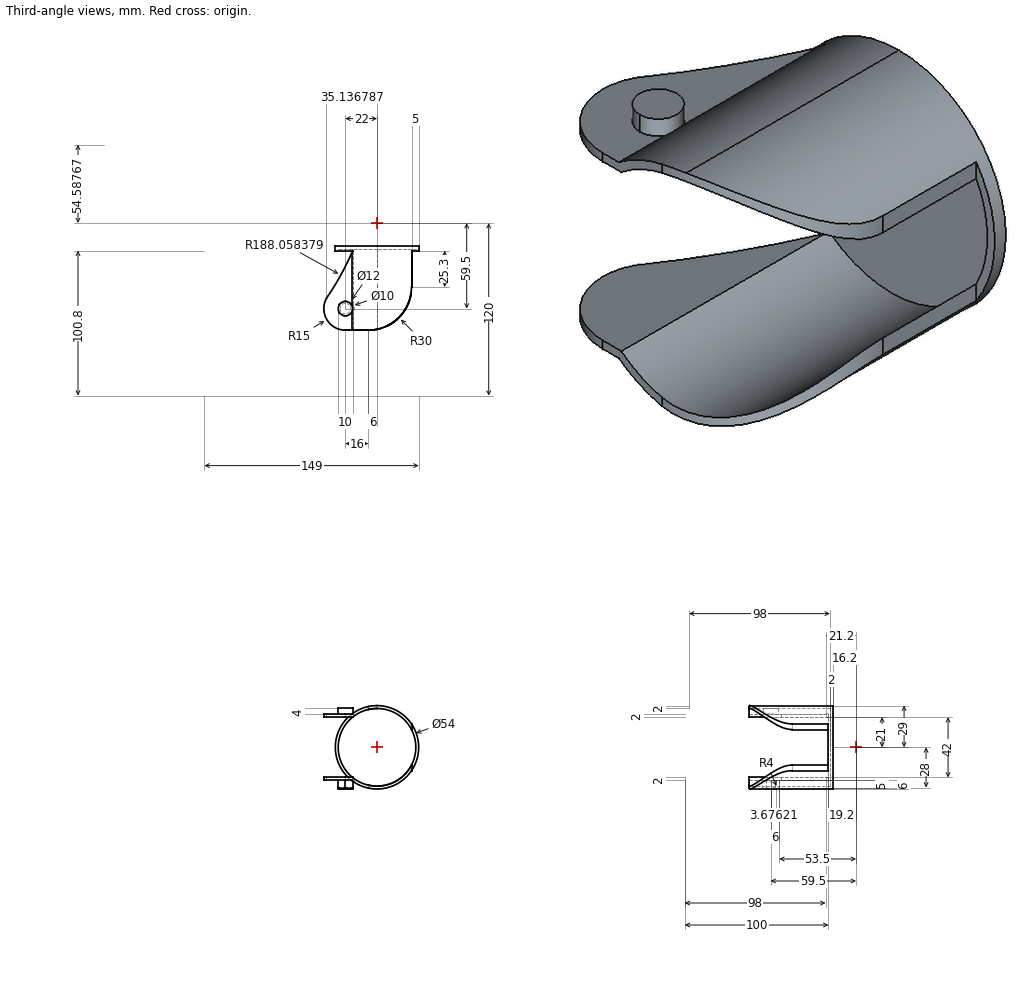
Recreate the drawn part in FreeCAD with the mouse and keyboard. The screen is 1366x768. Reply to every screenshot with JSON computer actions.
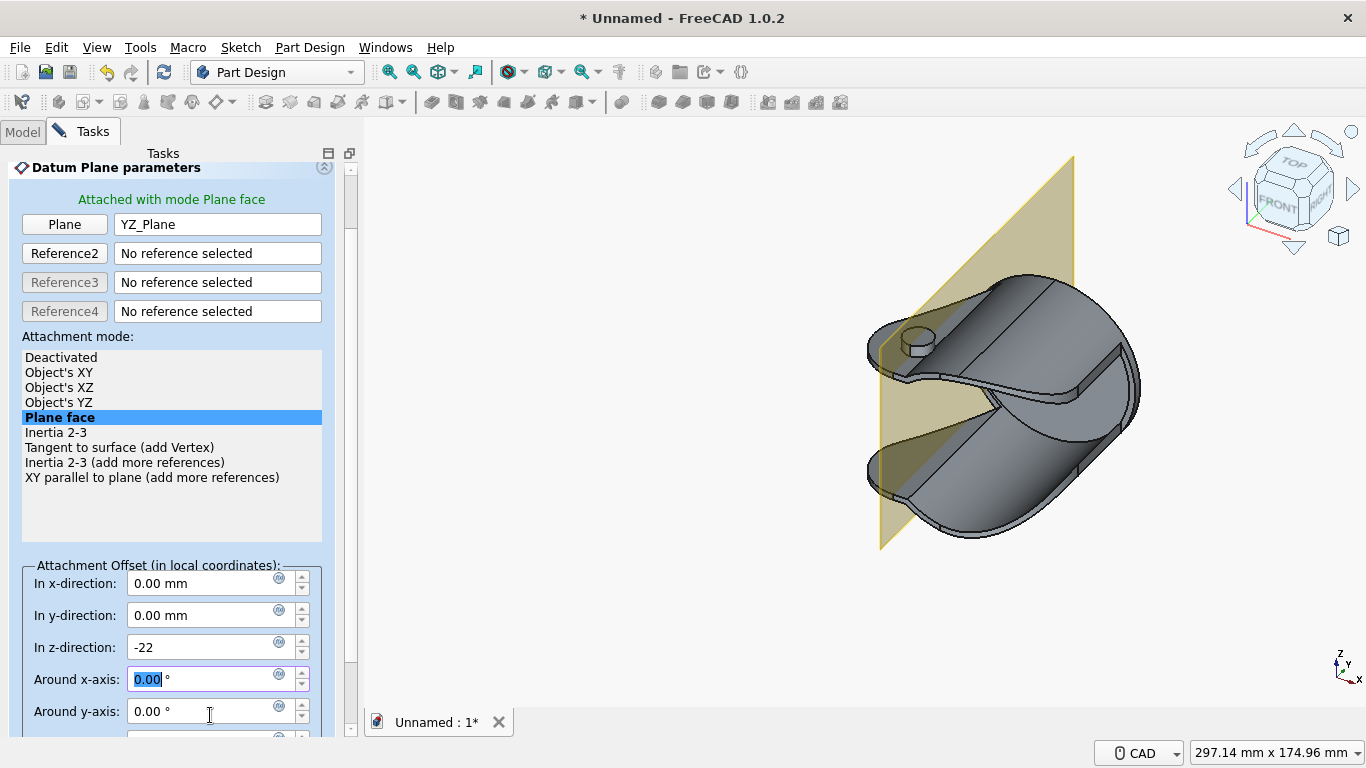
{"action": "scroll", "coordinate": [351, 450], "scroll_direction": "up", "scroll_amount": 2}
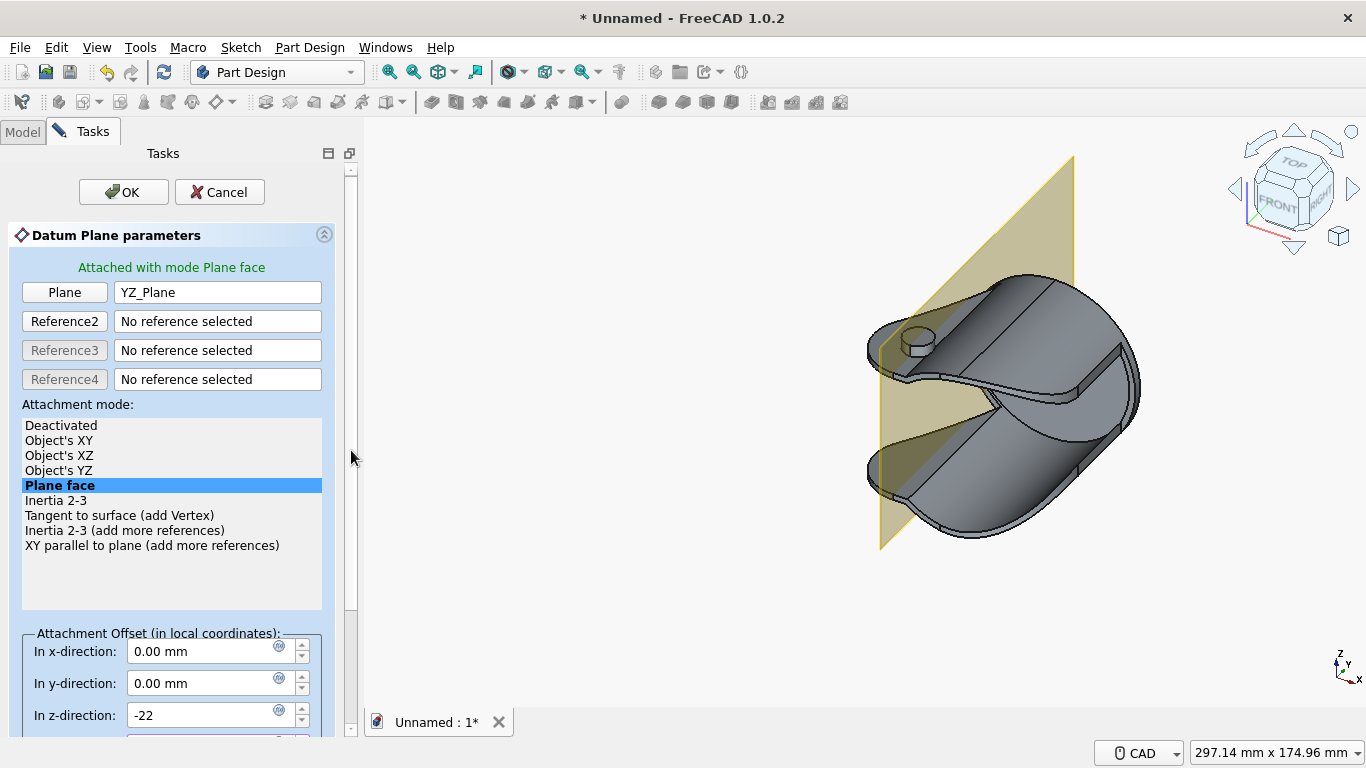
{"action": "left_click", "coordinate": [124, 192]}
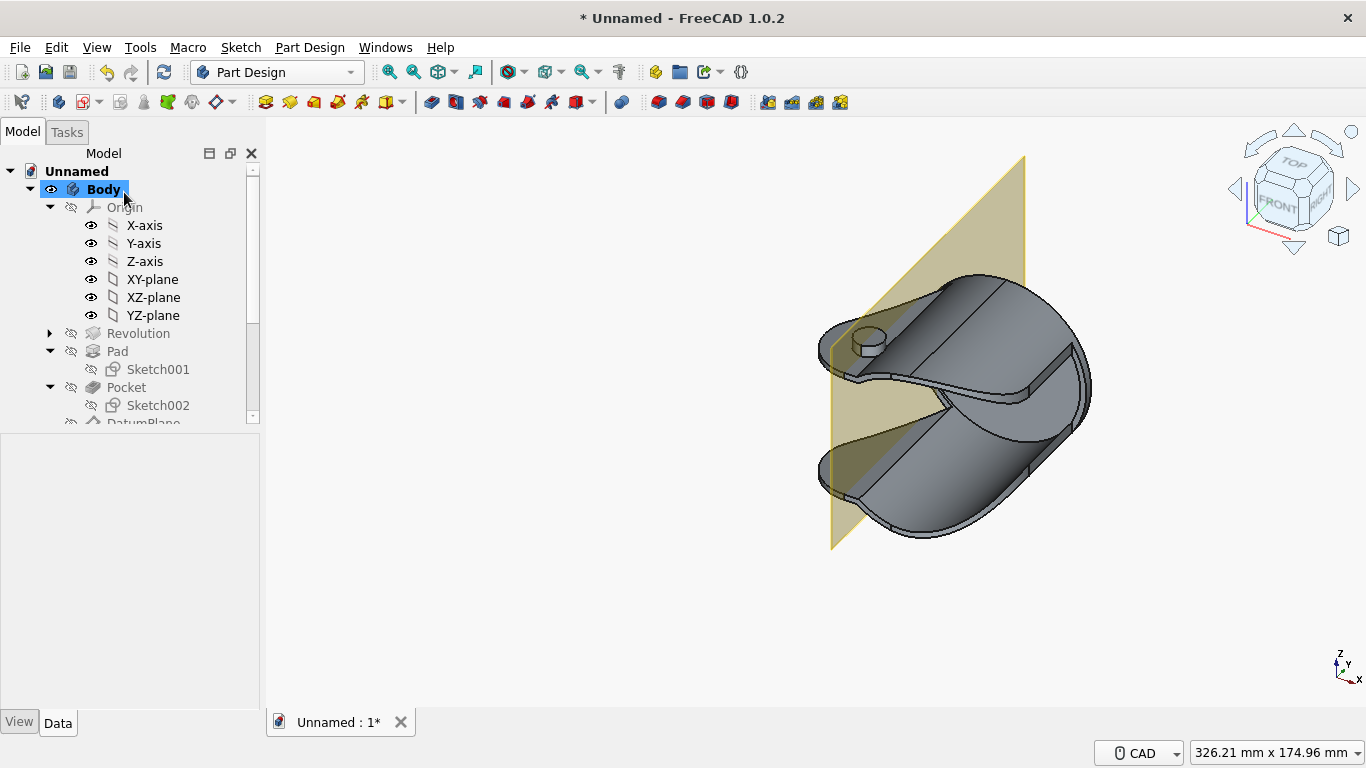
{"action": "scroll", "coordinate": [100, 293], "scroll_direction": "down", "scroll_amount": 3}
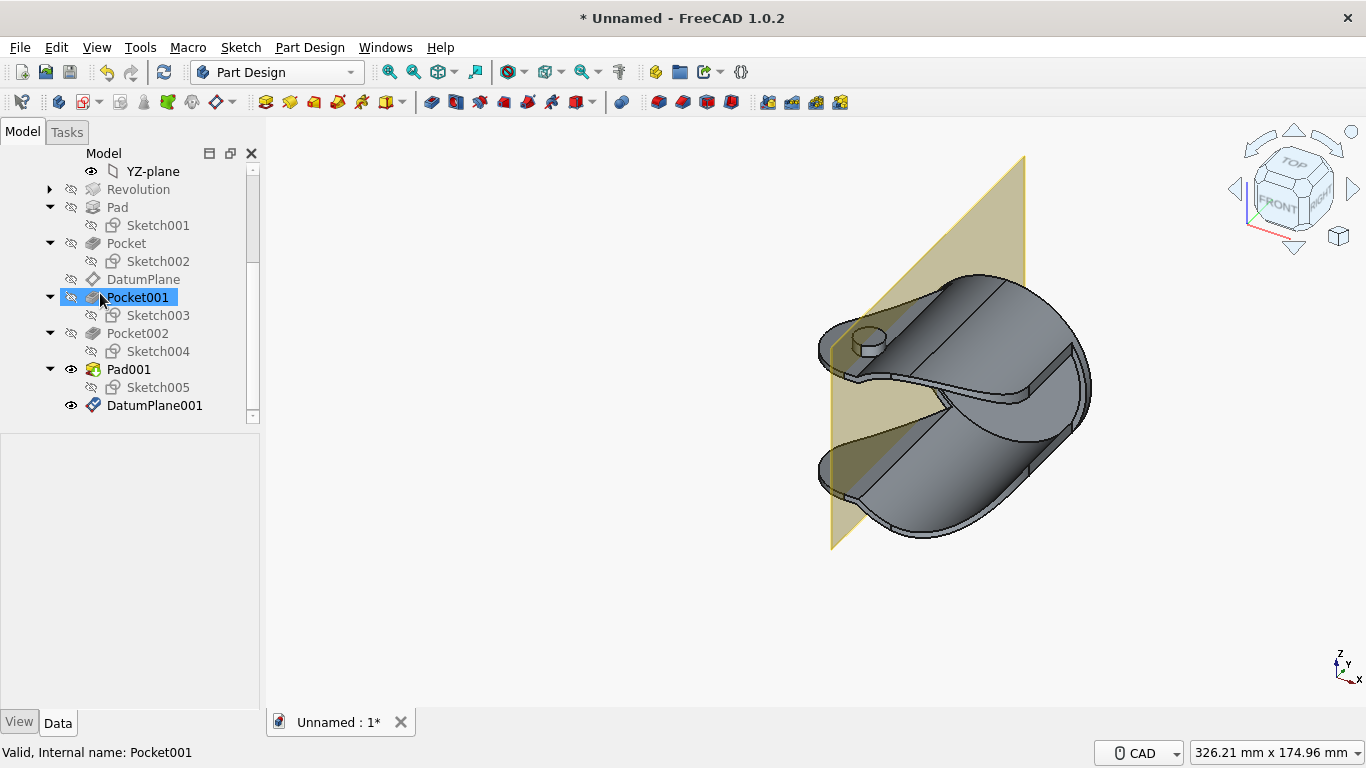
{"action": "left_click", "coordinate": [116, 405]}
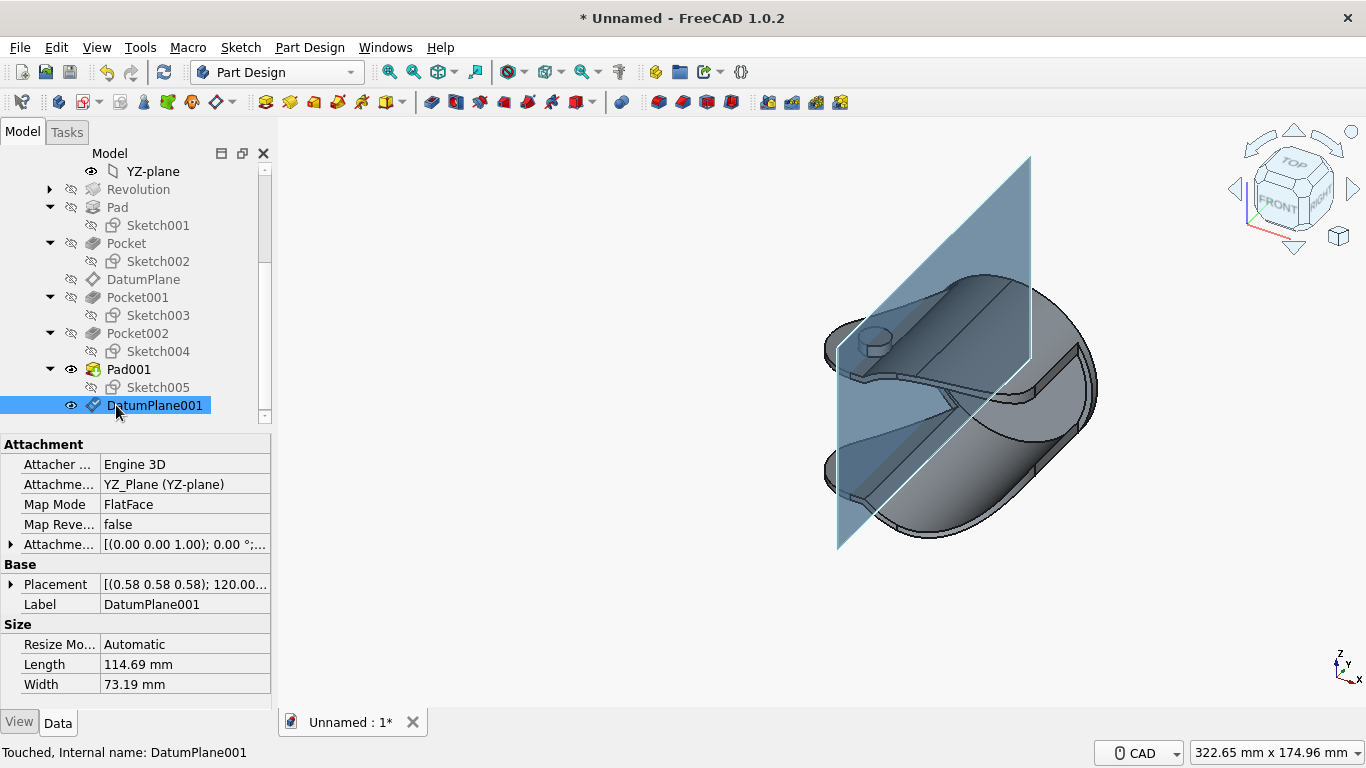
{"action": "left_click", "coordinate": [84, 102]}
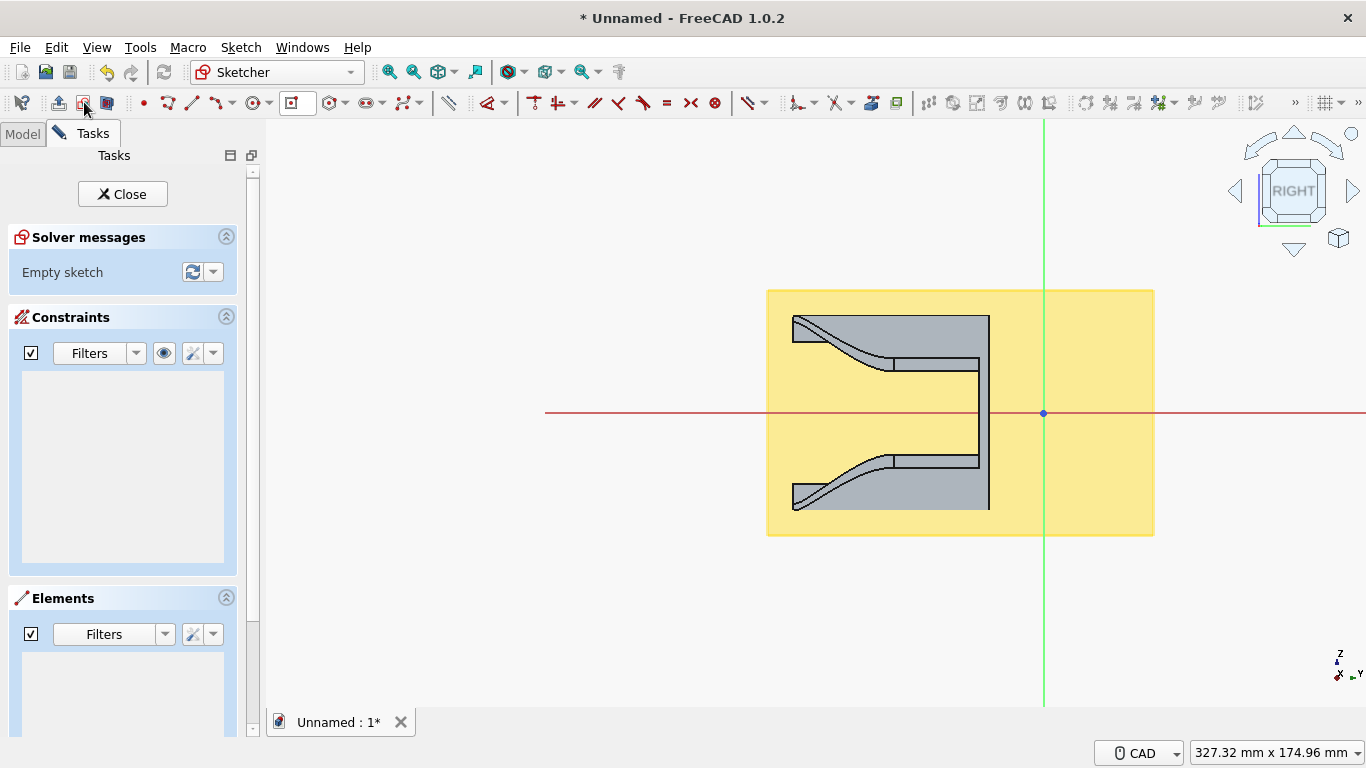
{"action": "left_click", "coordinate": [108, 104]}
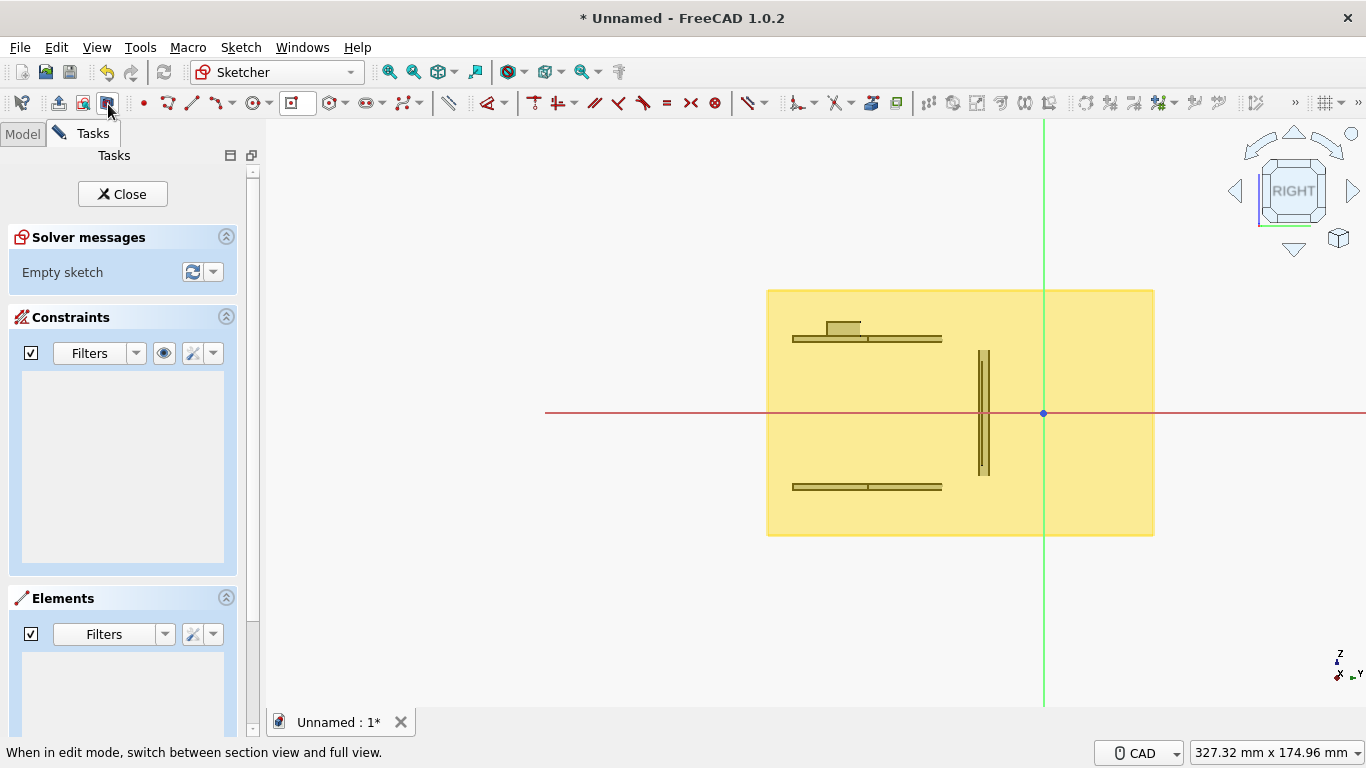
{"action": "scroll", "coordinate": [862, 503], "scroll_direction": "up", "scroll_amount": 13}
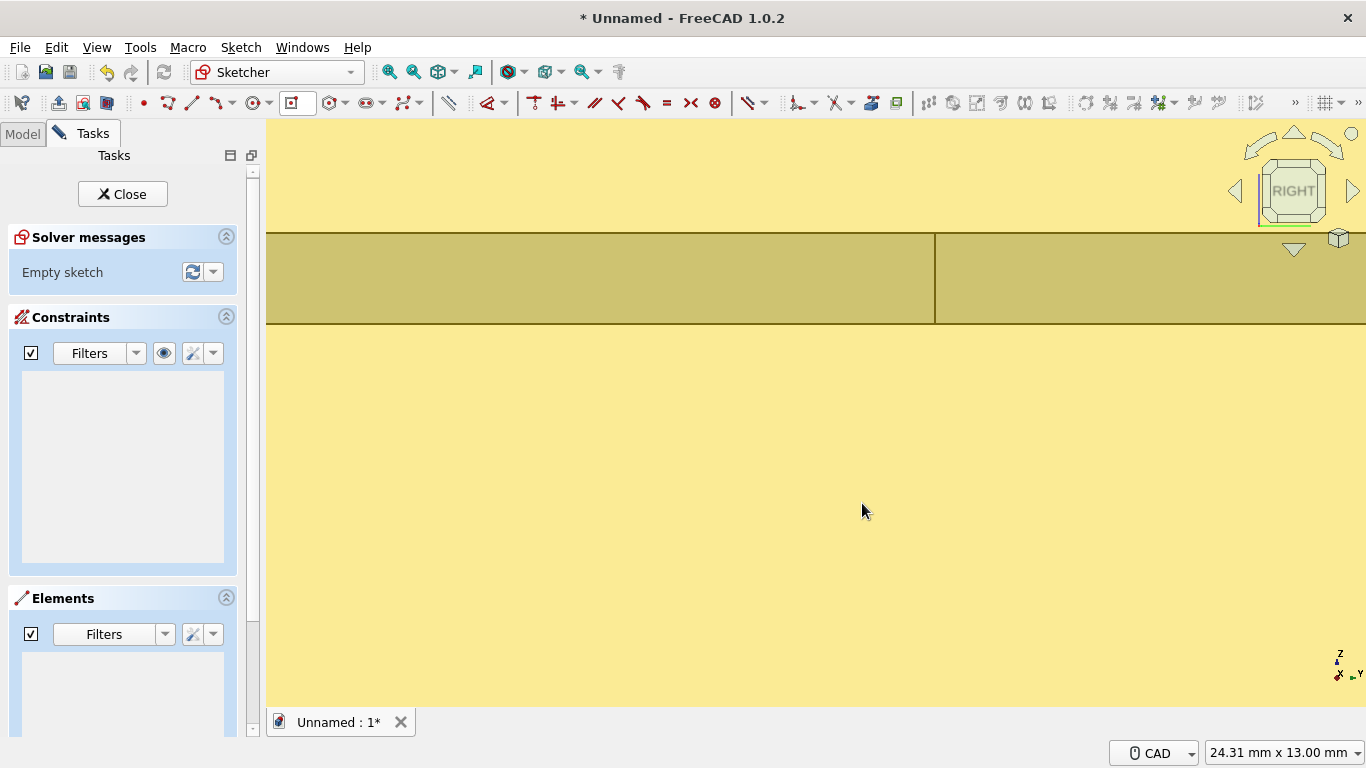
{"action": "left_click", "coordinate": [168, 104]}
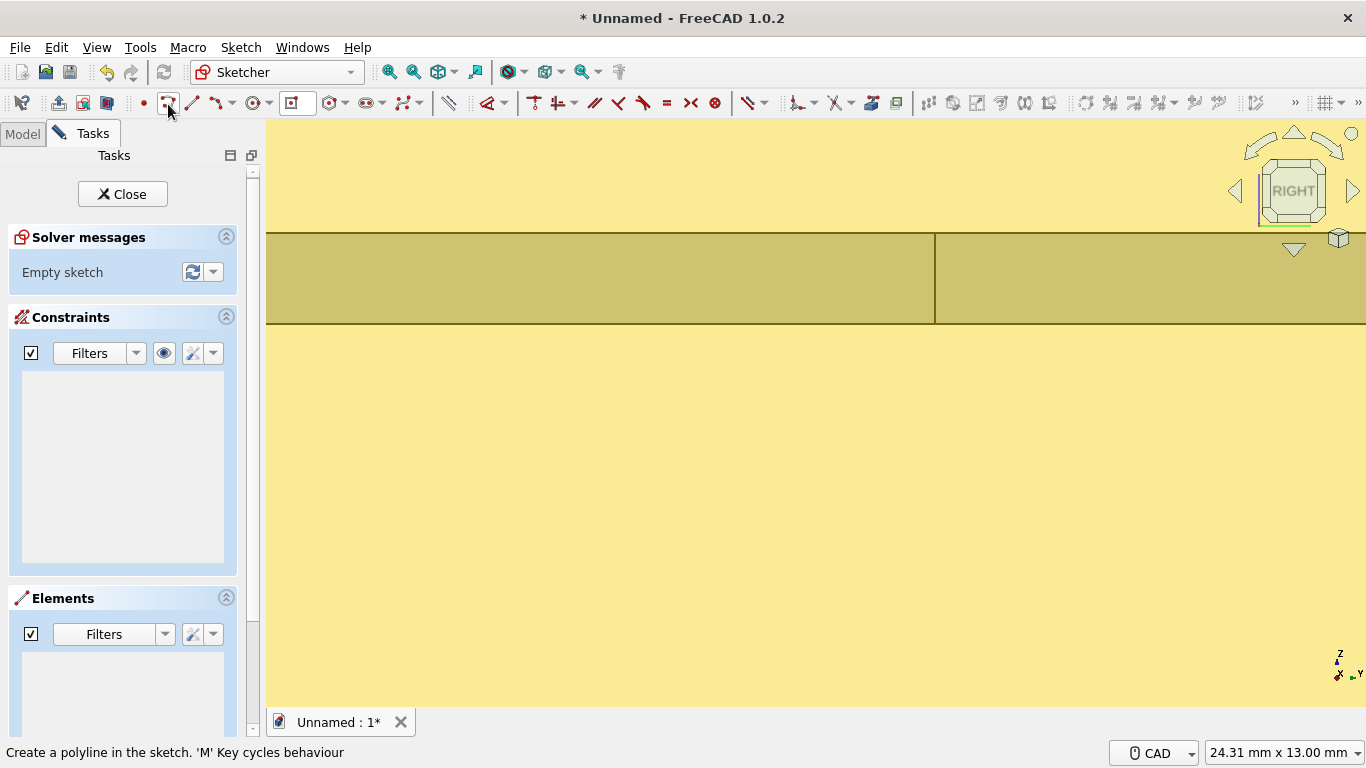
{"action": "left_click", "coordinate": [878, 550]}
{"action": "left_click", "coordinate": [878, 324]}
{"action": "left_click", "coordinate": [607, 324]}
{"action": "left_click", "coordinate": [607, 595]}
{"action": "left_click", "coordinate": [773, 595]}
{"action": "right_click", "coordinate": [773, 595]}